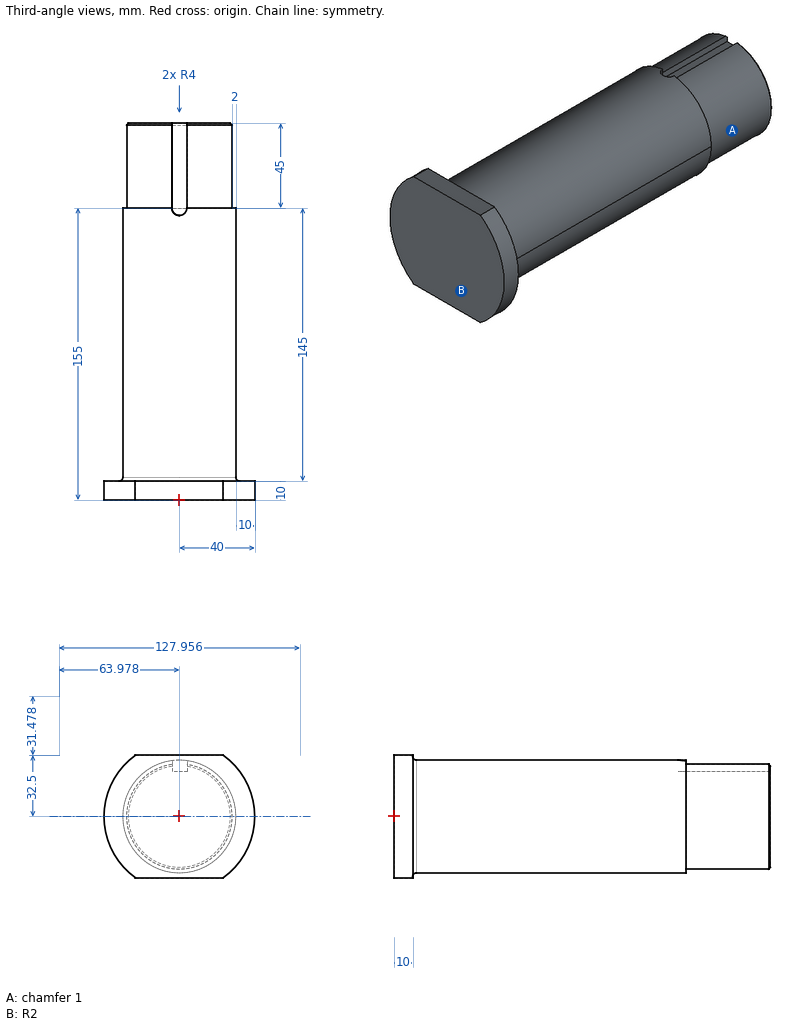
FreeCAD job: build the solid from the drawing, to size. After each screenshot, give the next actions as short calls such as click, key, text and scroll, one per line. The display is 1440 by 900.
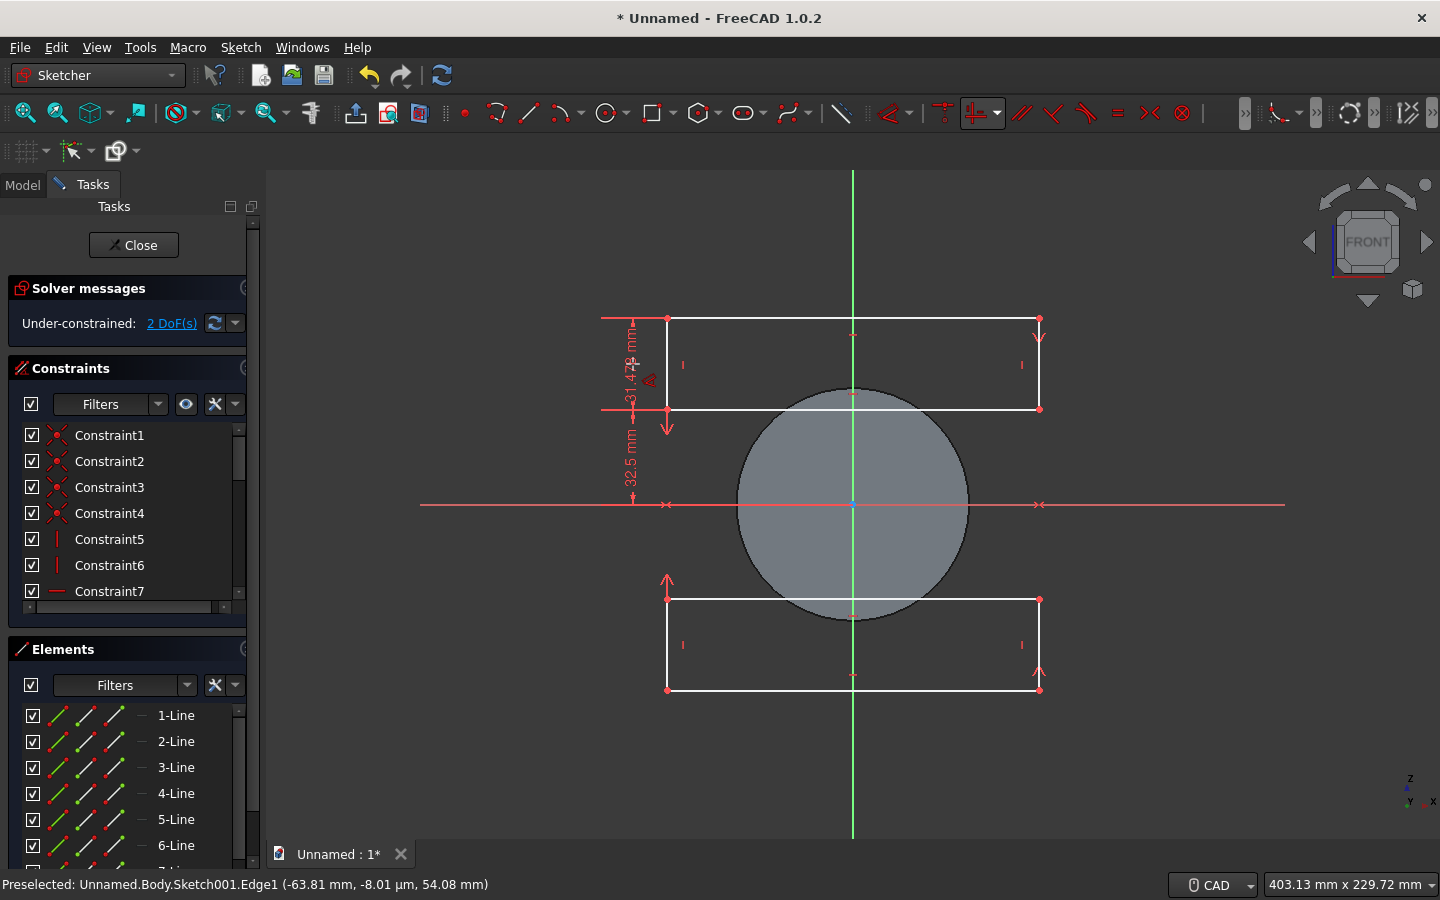
click(779, 410)
click(767, 376)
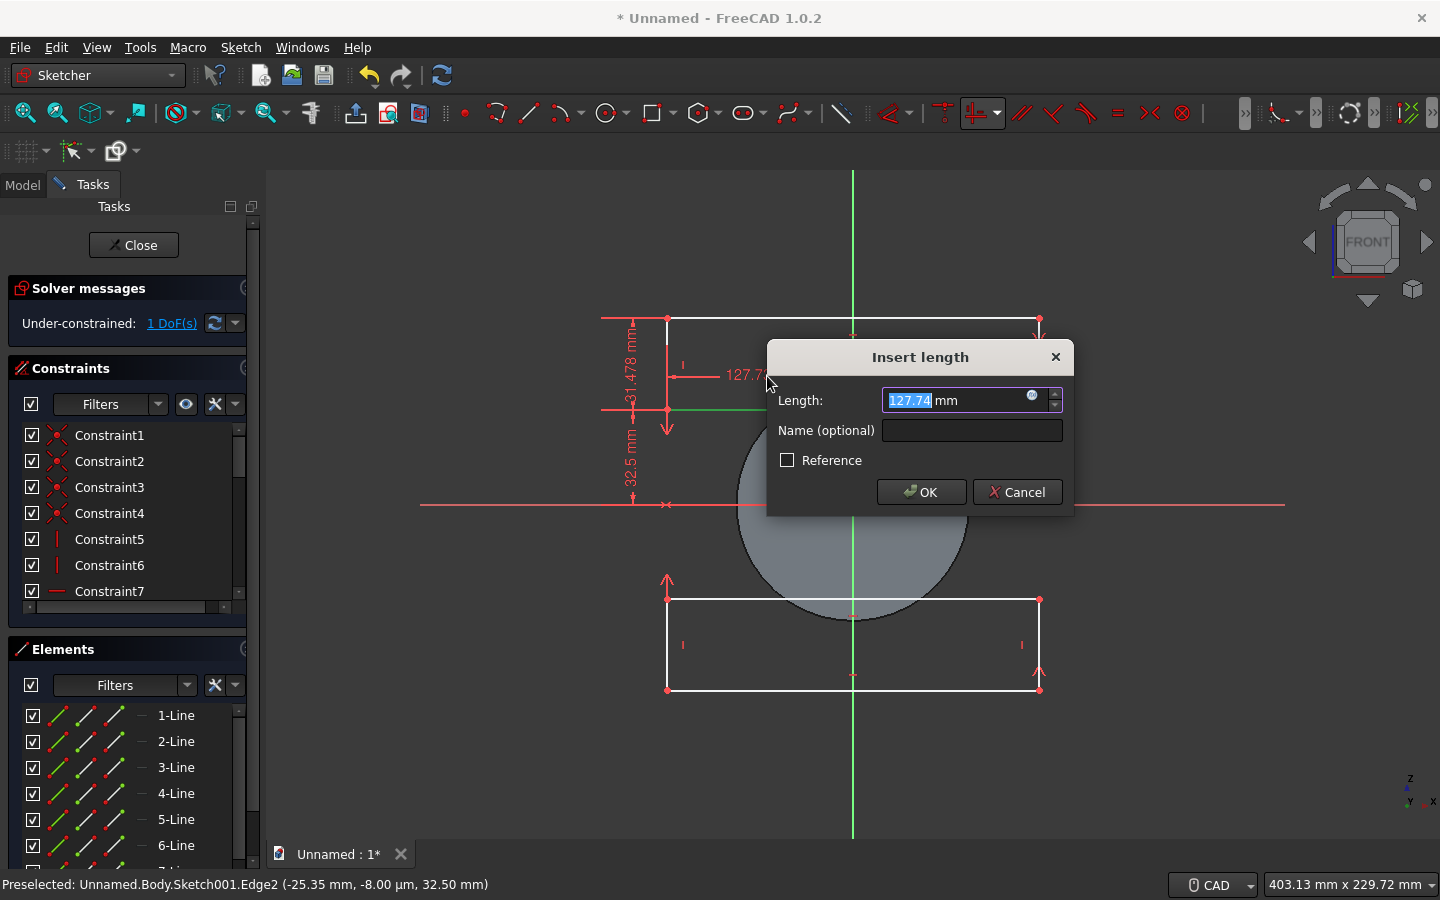
text(127.956)
key(Return)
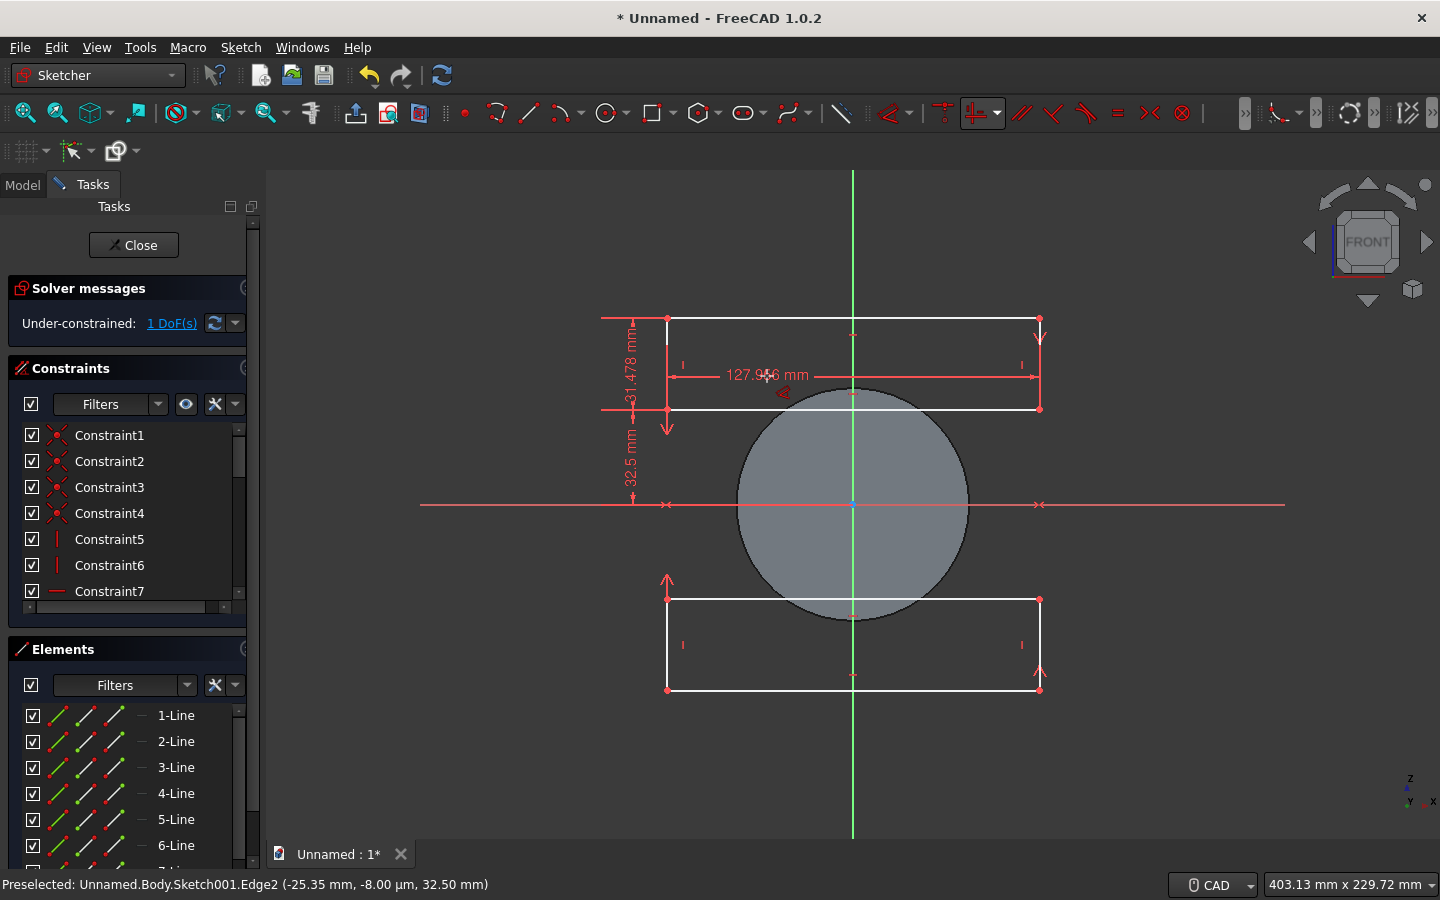
click(667, 318)
click(760, 284)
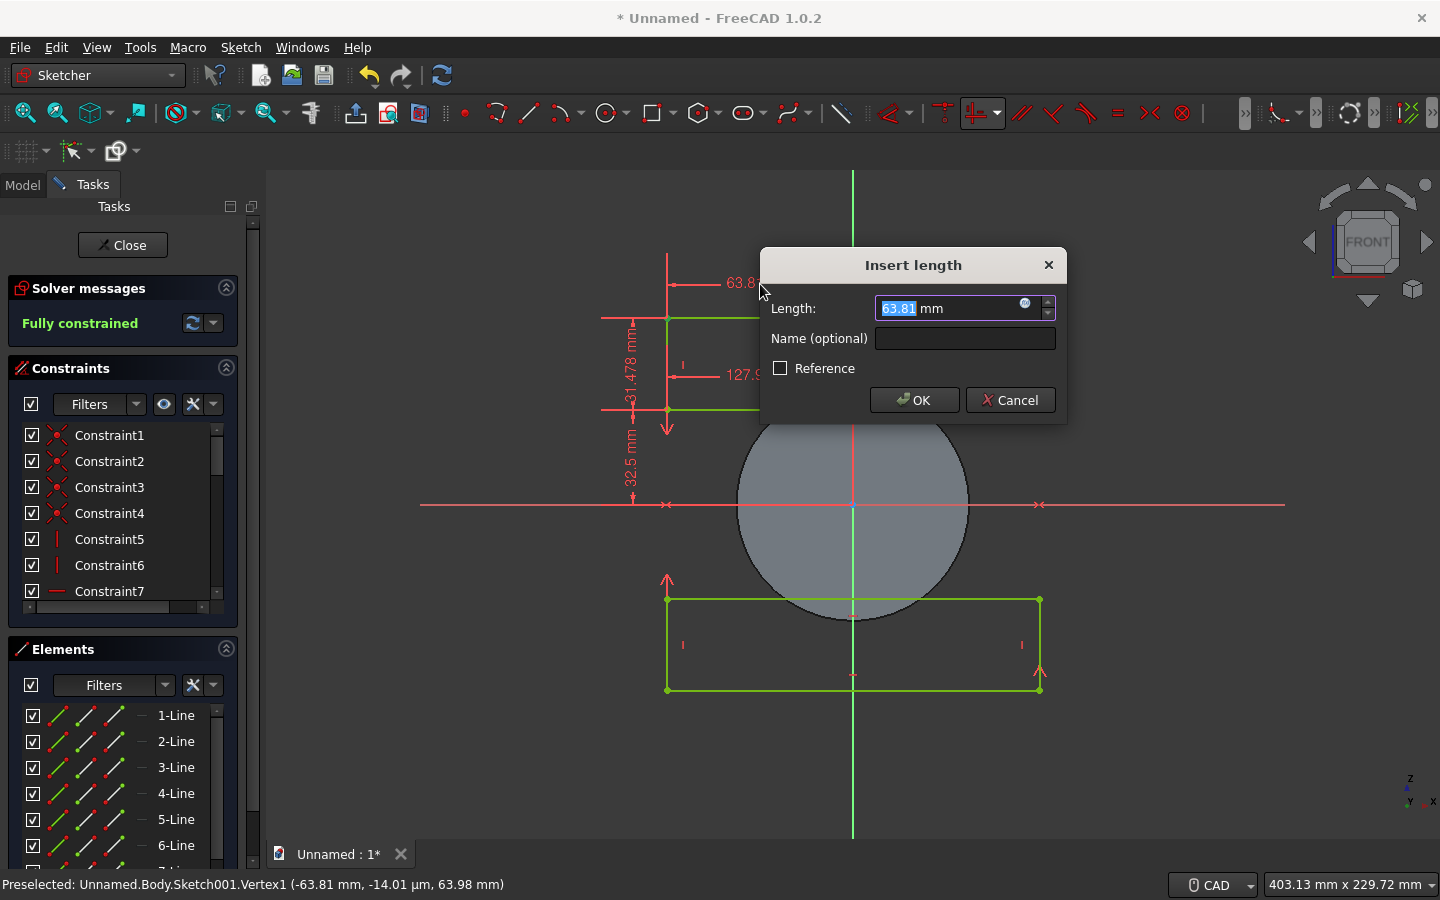
text(63.978)
key(Return)
key(Escape)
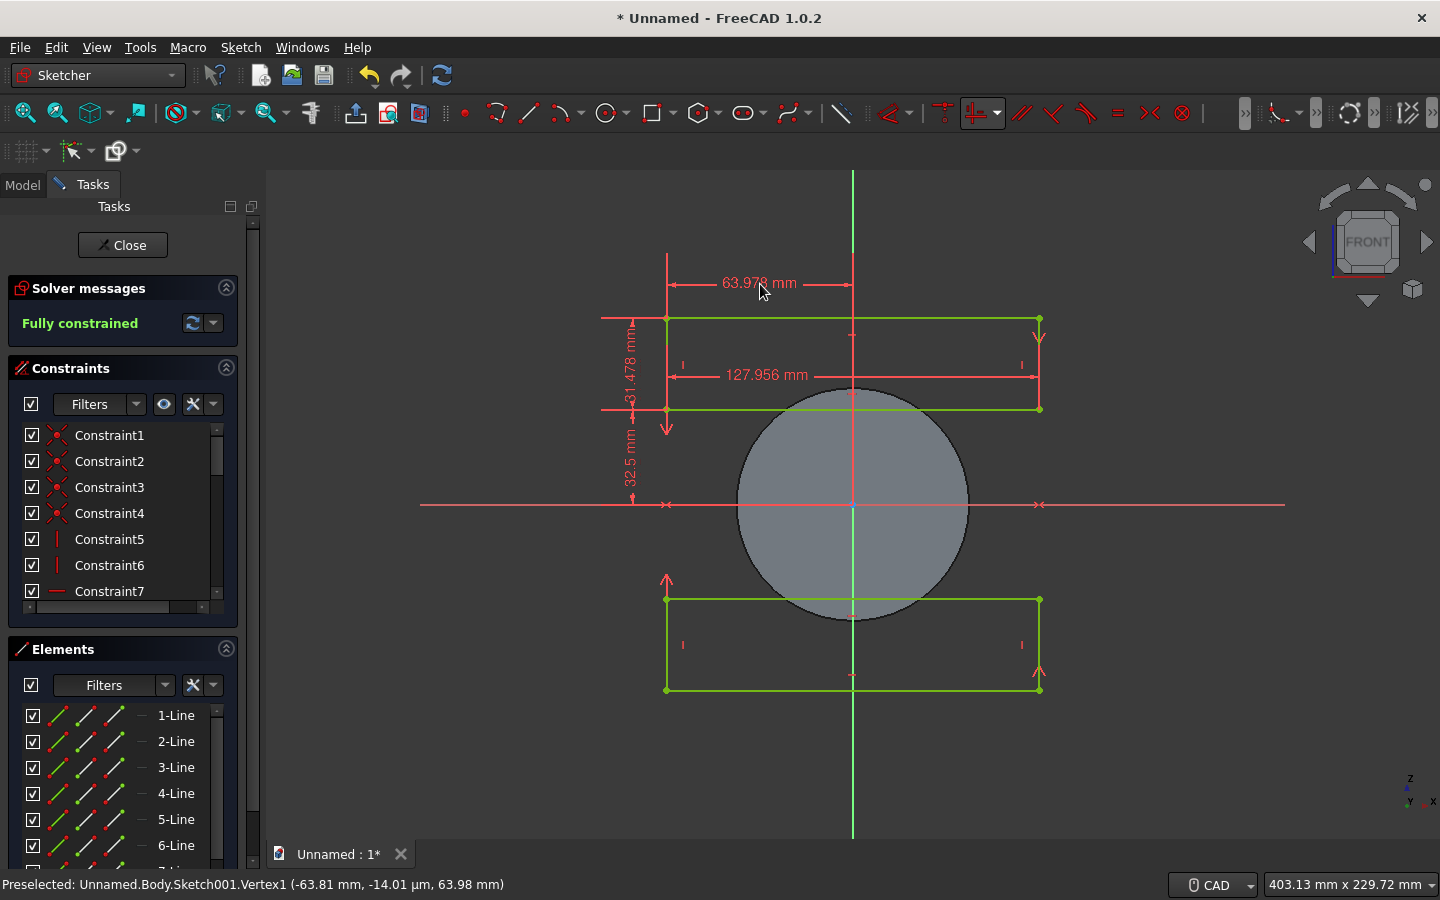
click(123, 245)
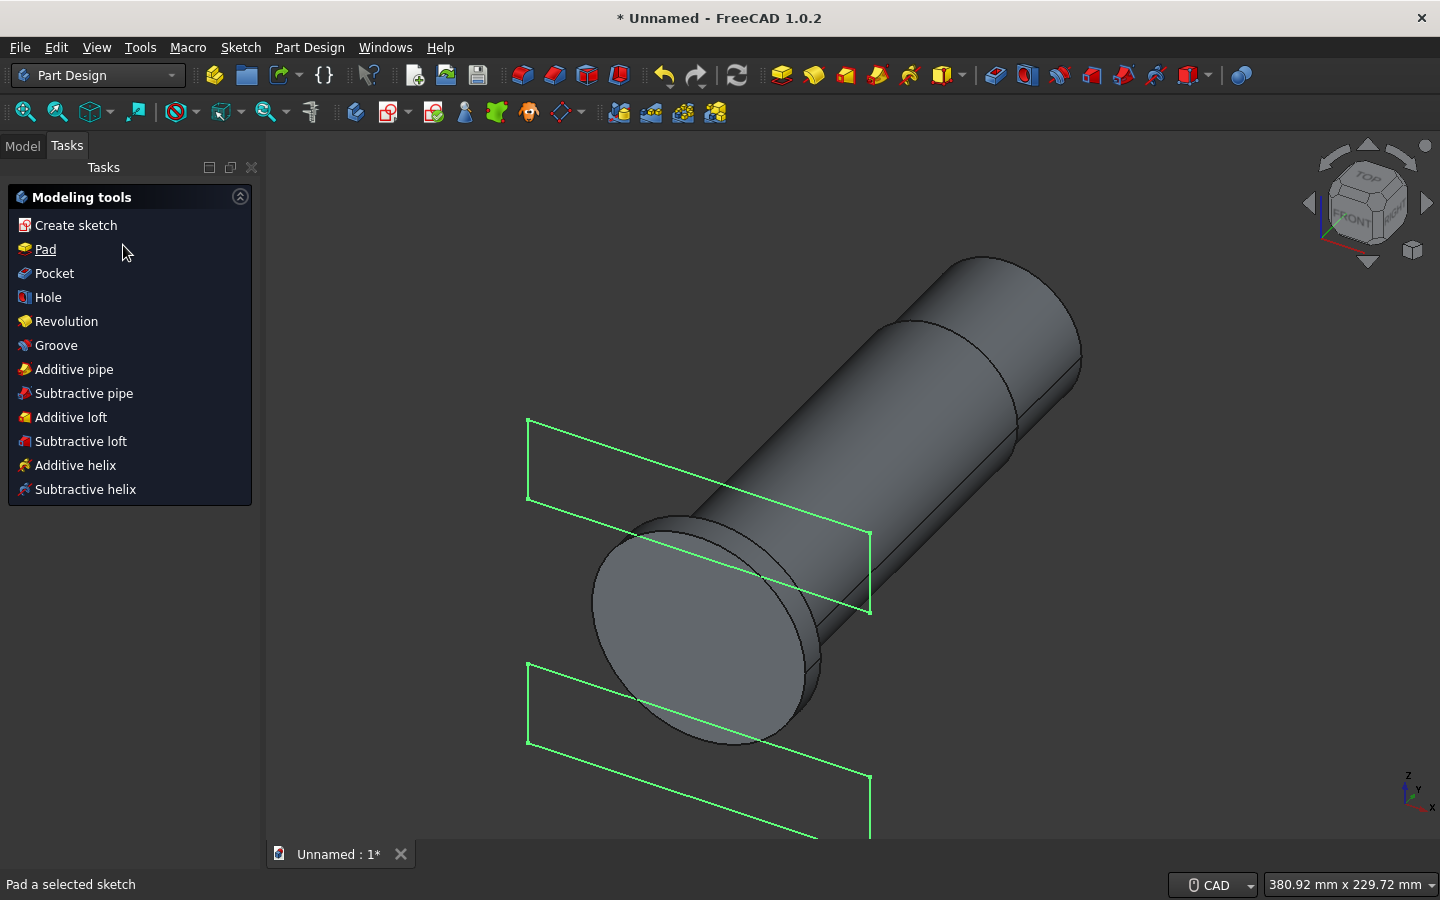
click(996, 76)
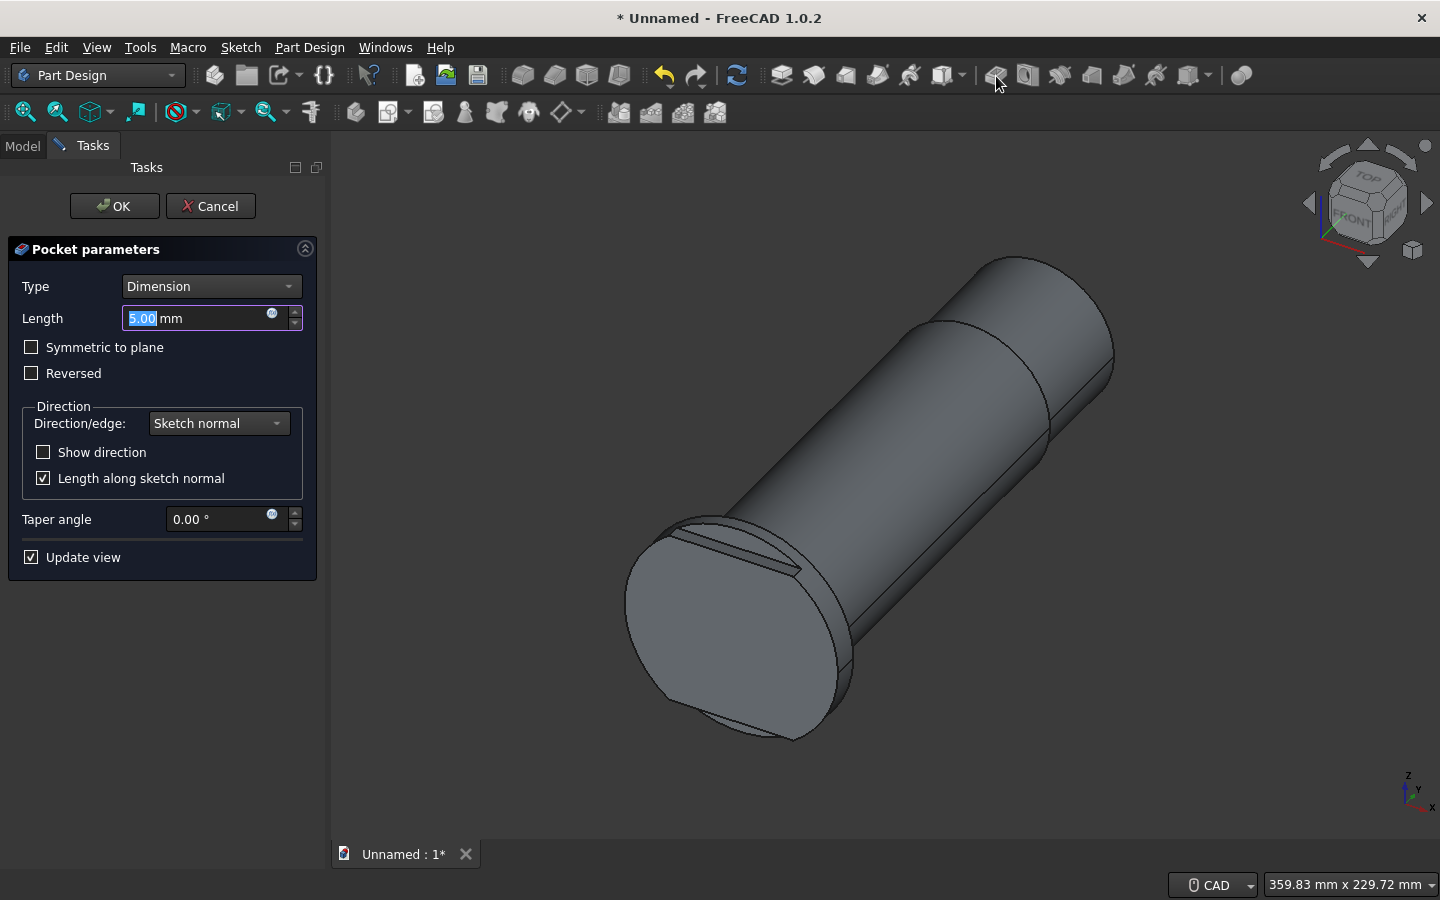
text(10)
key(Tab)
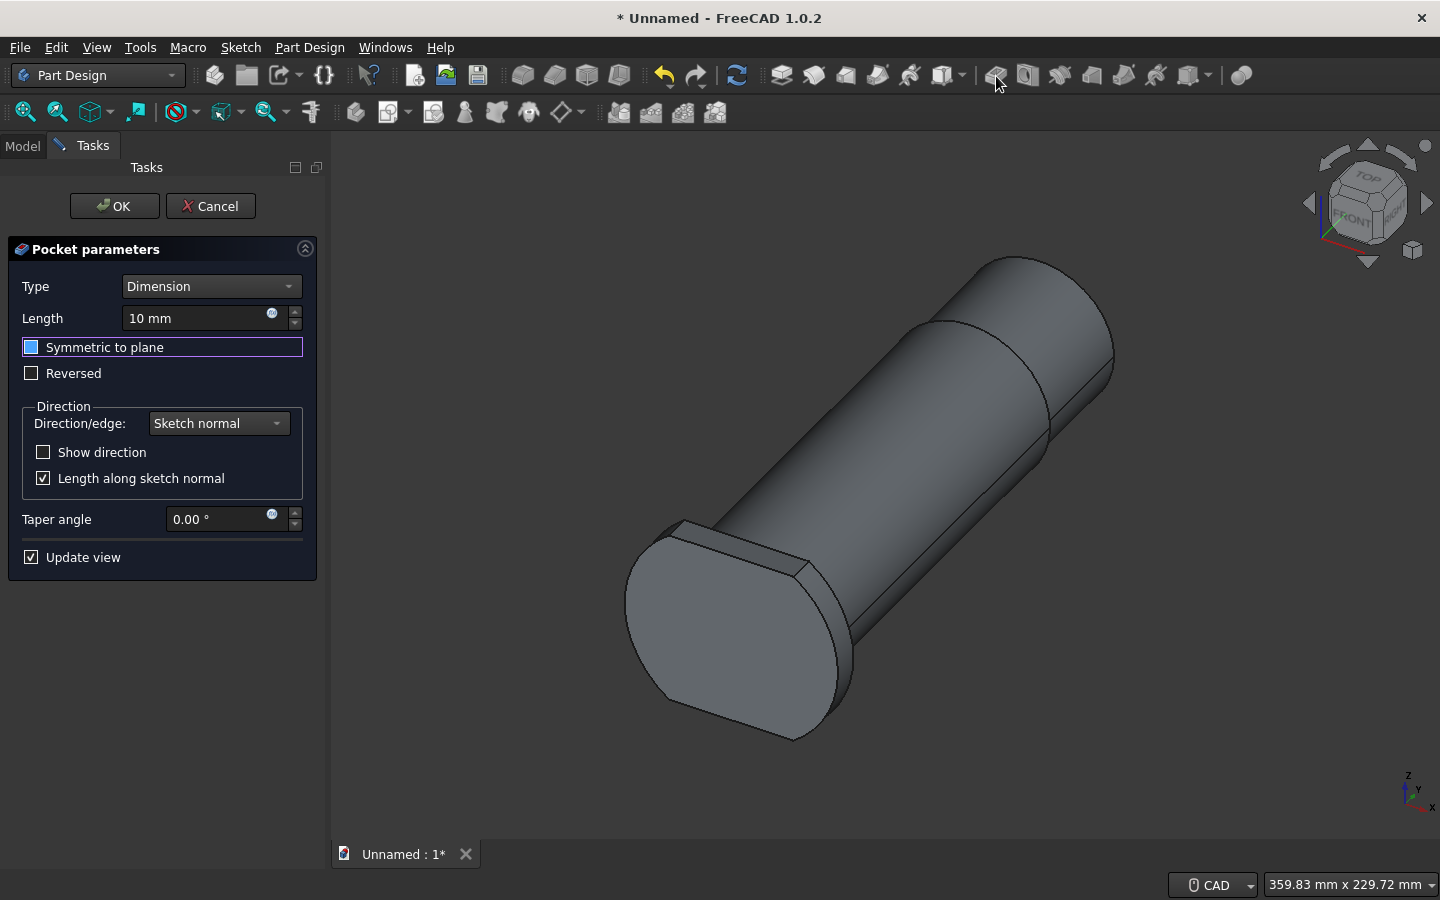
click(115, 206)